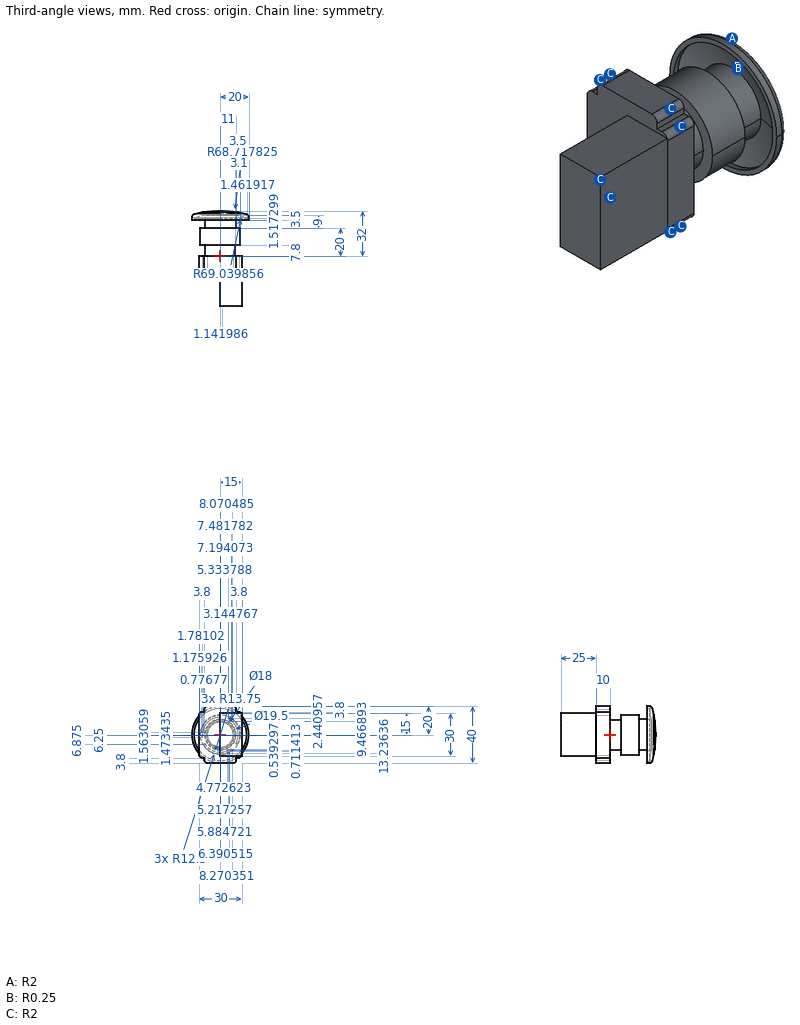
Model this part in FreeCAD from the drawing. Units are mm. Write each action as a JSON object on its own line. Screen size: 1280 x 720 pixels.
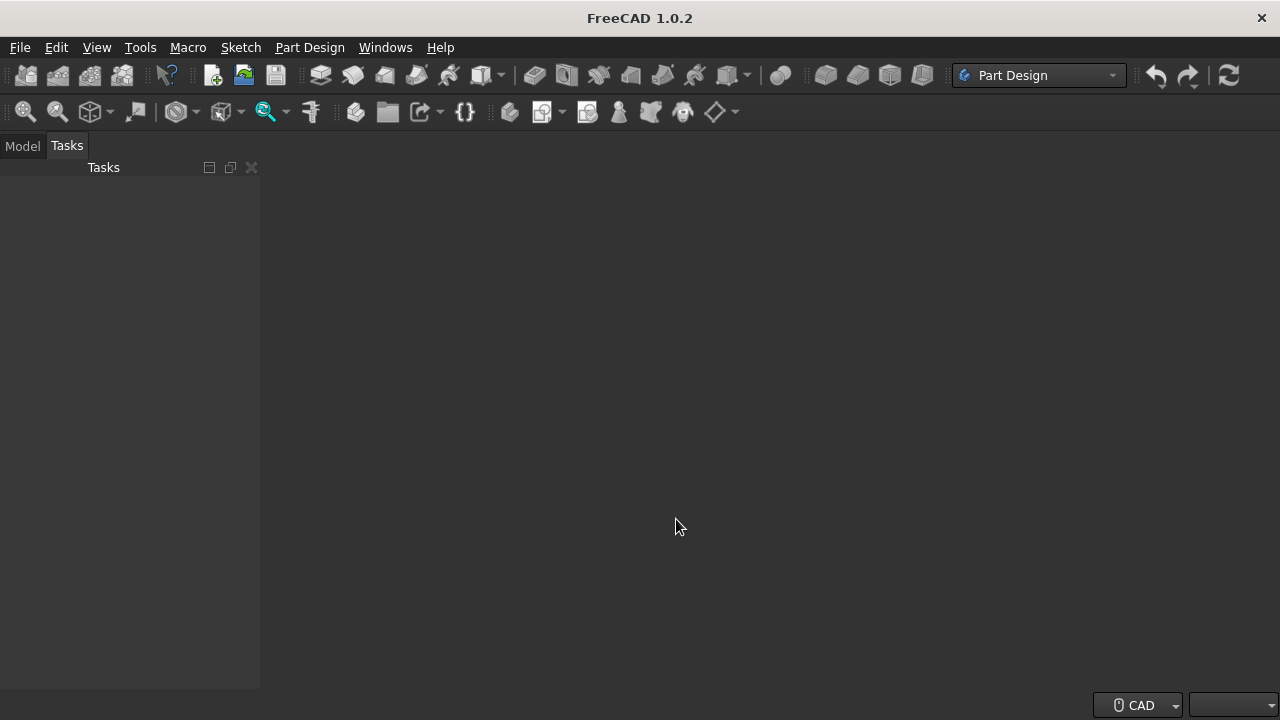
{"action": "left_click", "coordinate": [212, 76]}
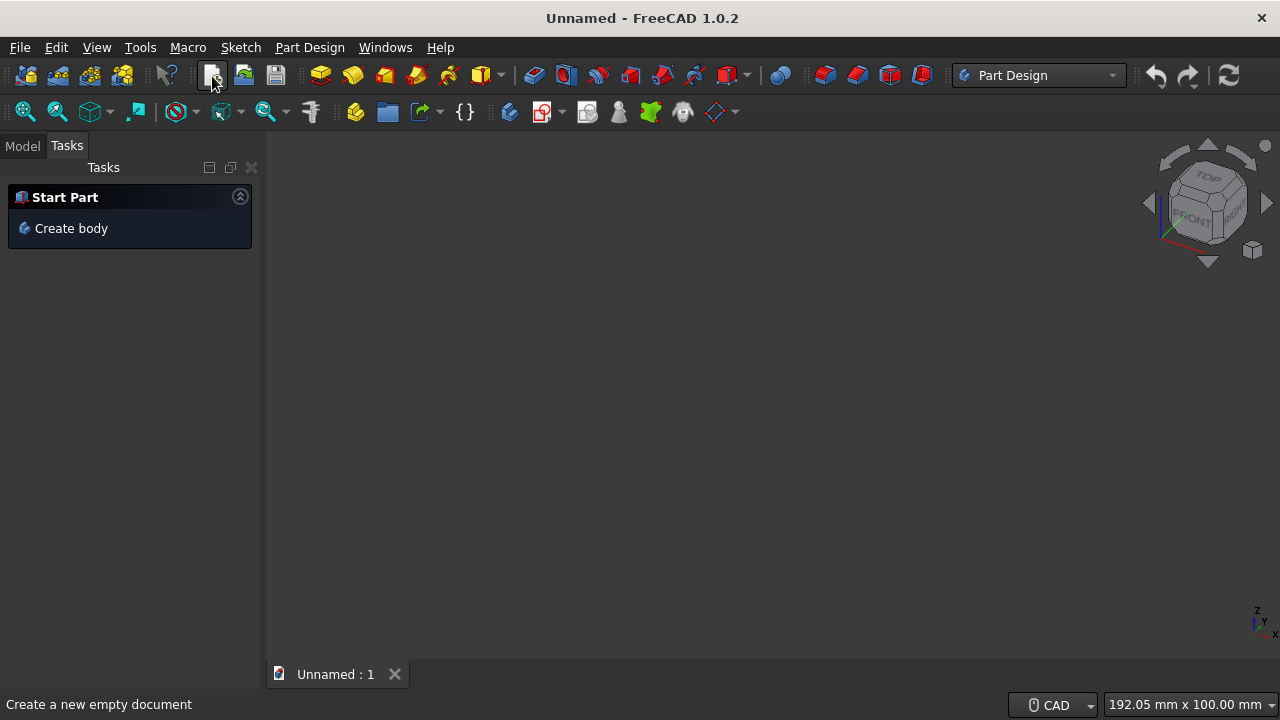
{"action": "left_click", "coordinate": [542, 112]}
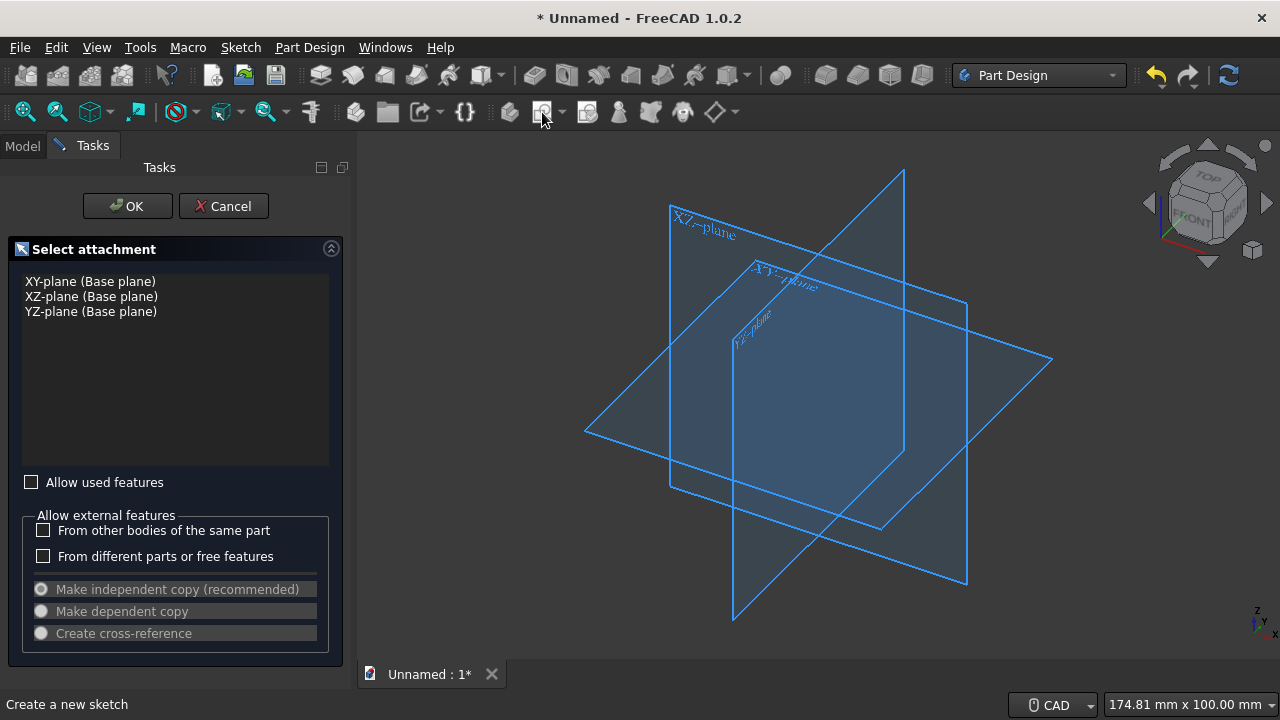
{"action": "left_click", "coordinate": [82, 282]}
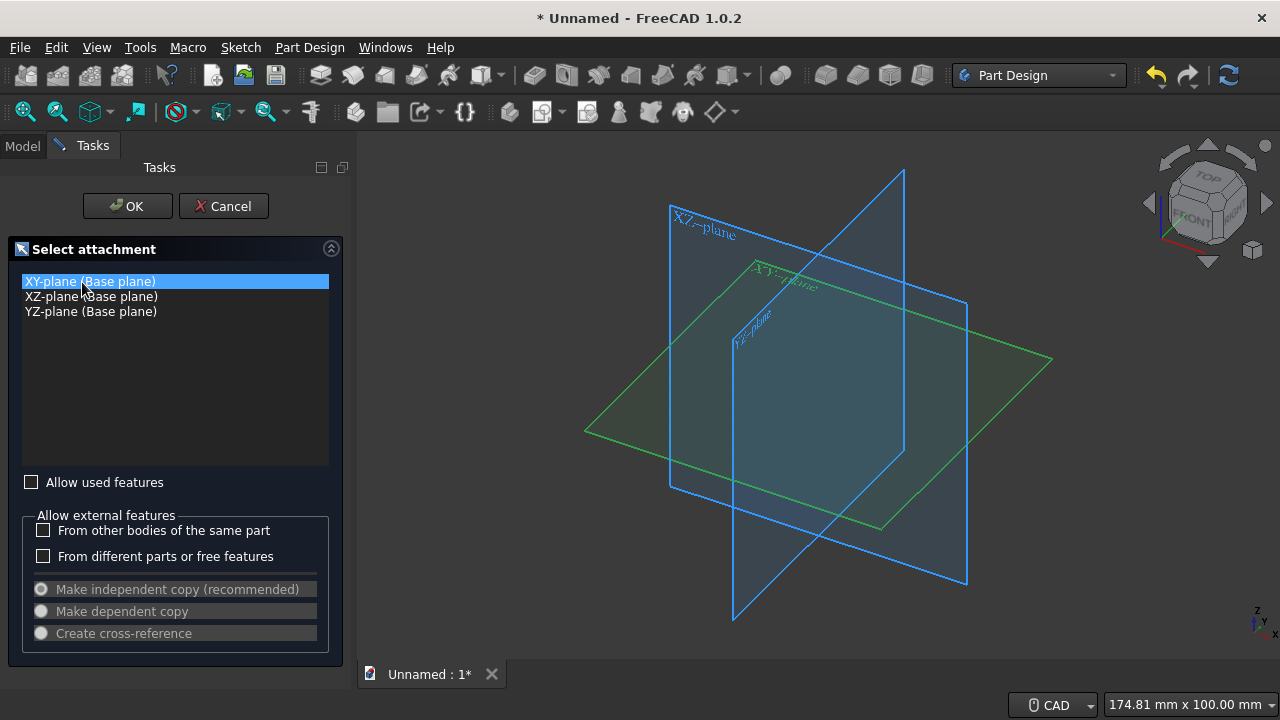
{"action": "left_click", "coordinate": [128, 206]}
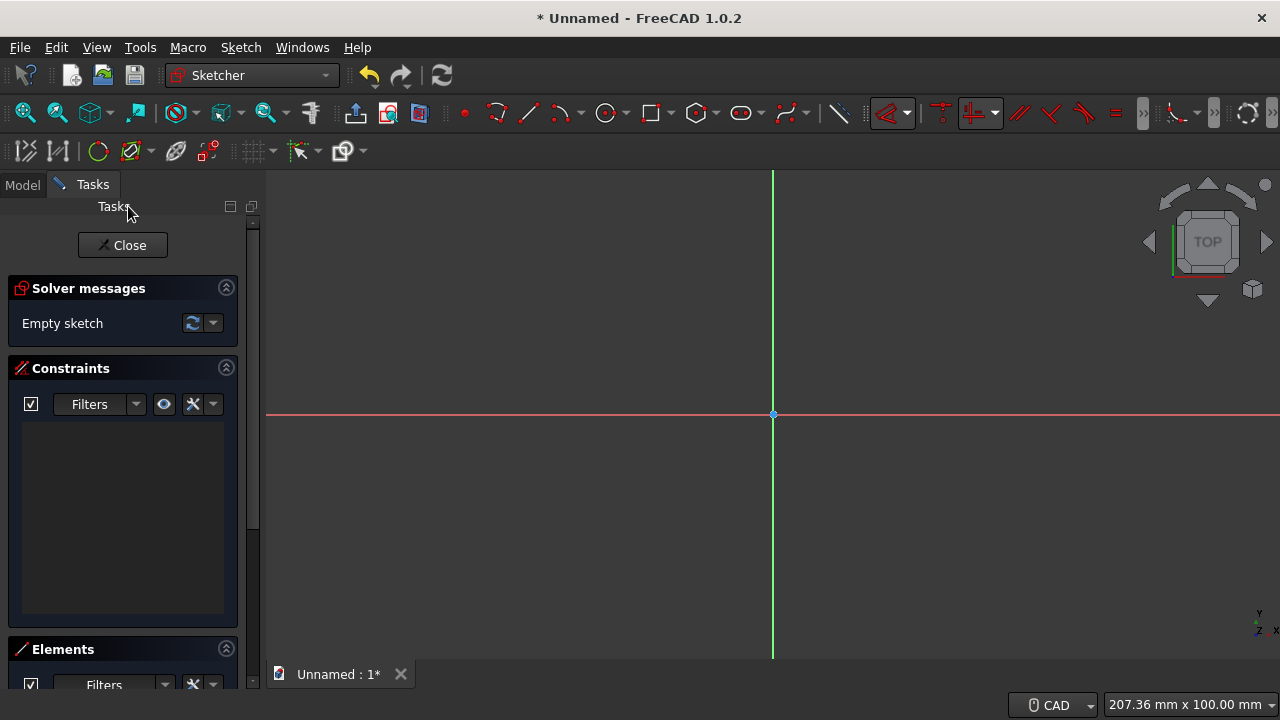
{"action": "scroll", "coordinate": [965, 241], "scroll_direction": "up", "scroll_amount": 3}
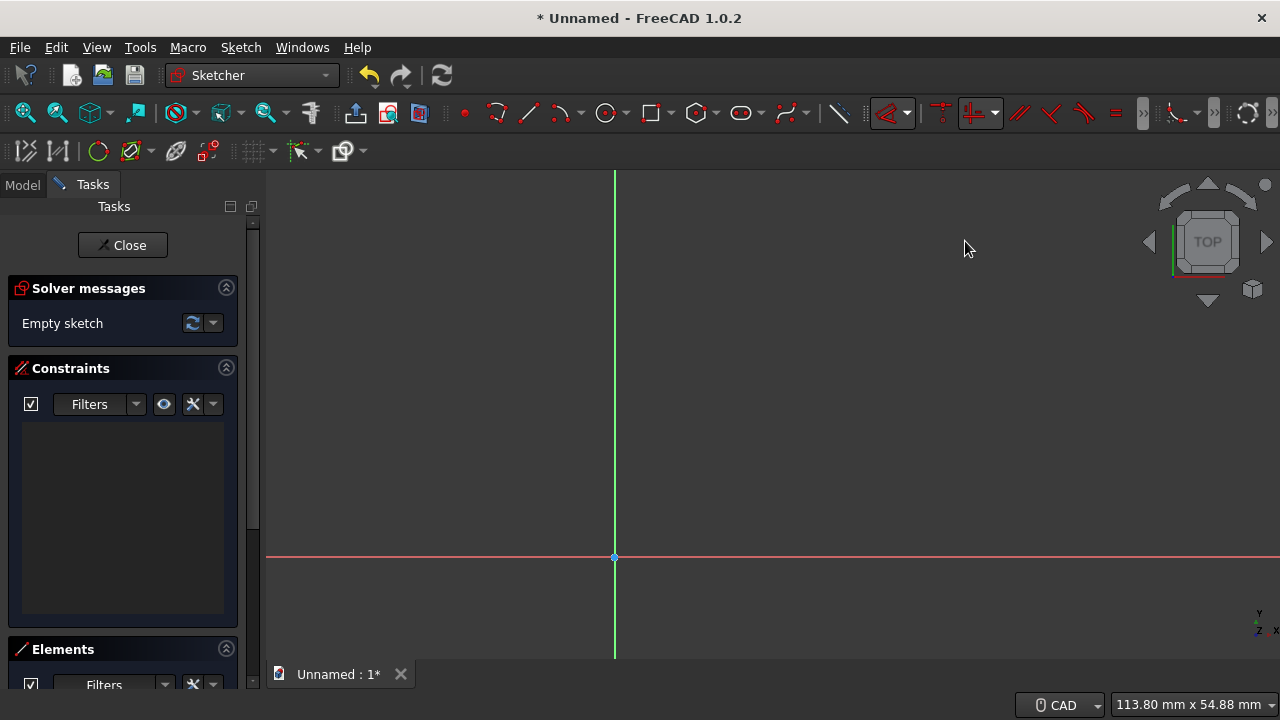
{"action": "left_click", "coordinate": [498, 114]}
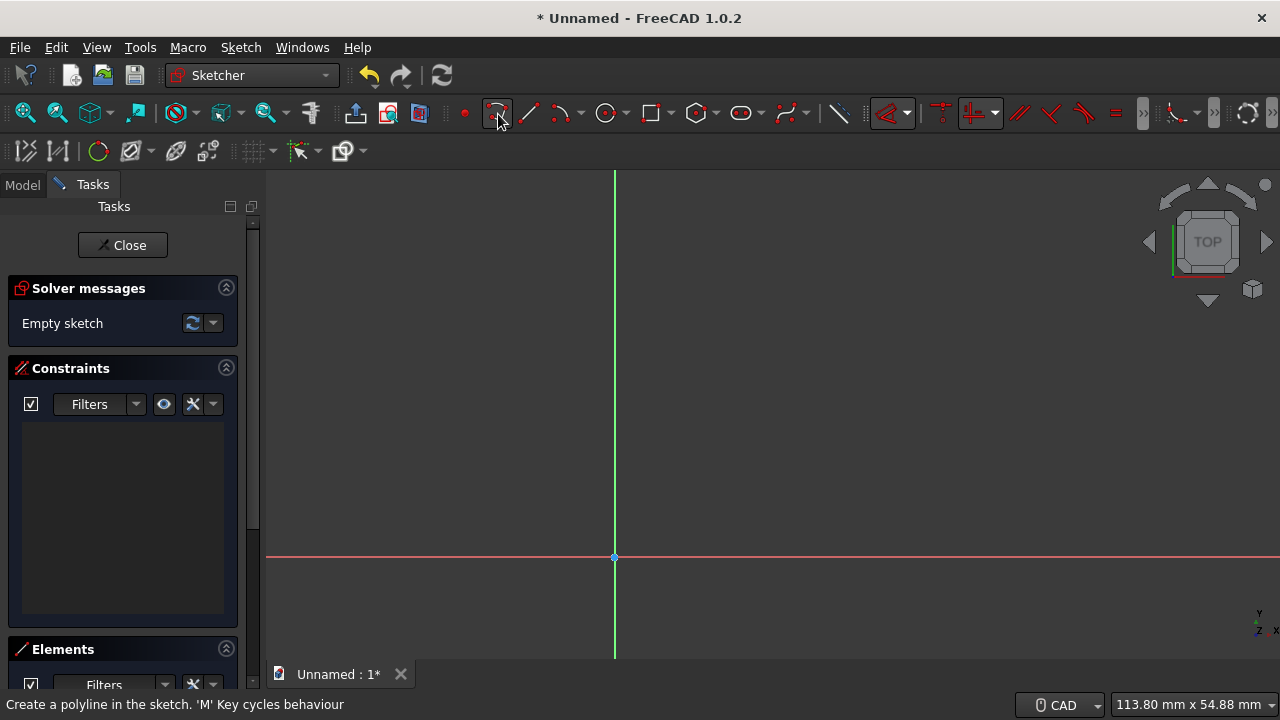
{"action": "left_click", "coordinate": [780, 313]}
{"action": "left_click", "coordinate": [780, 327]}
{"action": "left_click", "coordinate": [793, 327]}
{"action": "left_click", "coordinate": [793, 295]}
{"action": "right_click", "coordinate": [793, 295]}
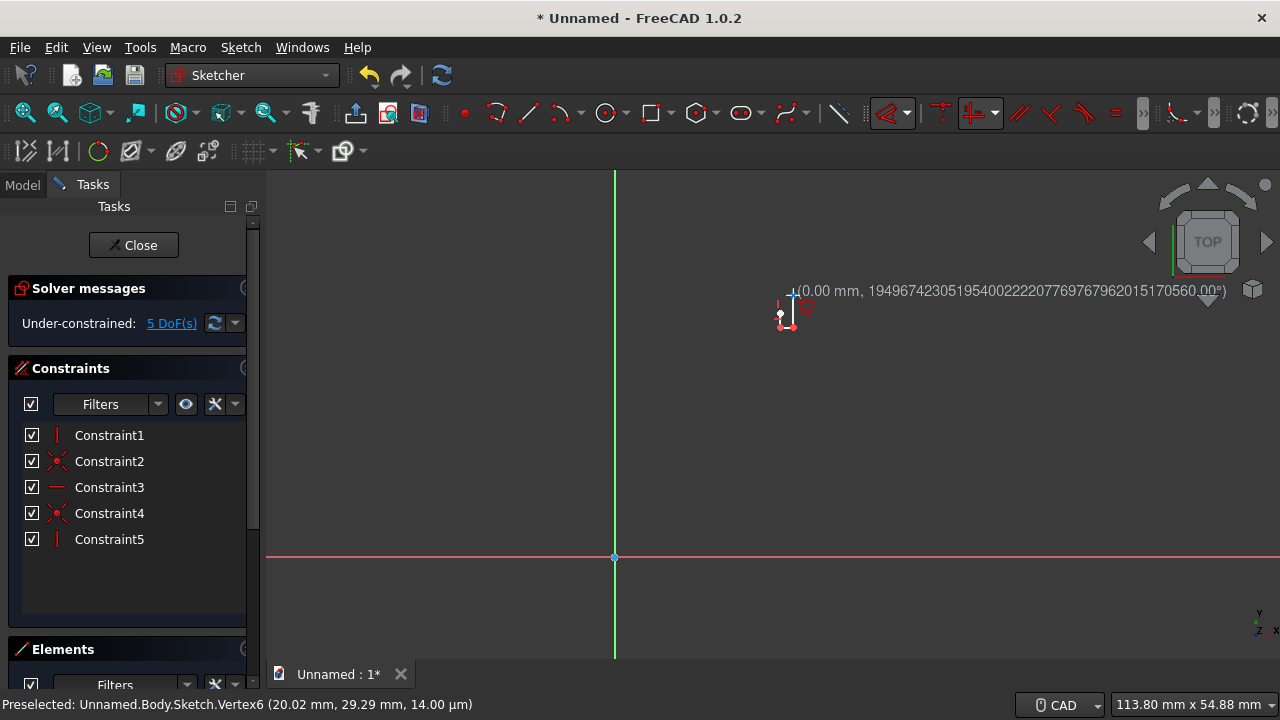
{"action": "left_click", "coordinate": [615, 272]}
{"action": "left_click", "coordinate": [615, 557]}
{"action": "left_click", "coordinate": [709, 548]}
{"action": "left_click", "coordinate": [709, 488]}
{"action": "left_click", "coordinate": [740, 488]}
{"action": "left_click", "coordinate": [740, 379]}
{"action": "left_click", "coordinate": [713, 379]}
{"action": "left_click", "coordinate": [713, 299]}
{"action": "right_click", "coordinate": [713, 299]}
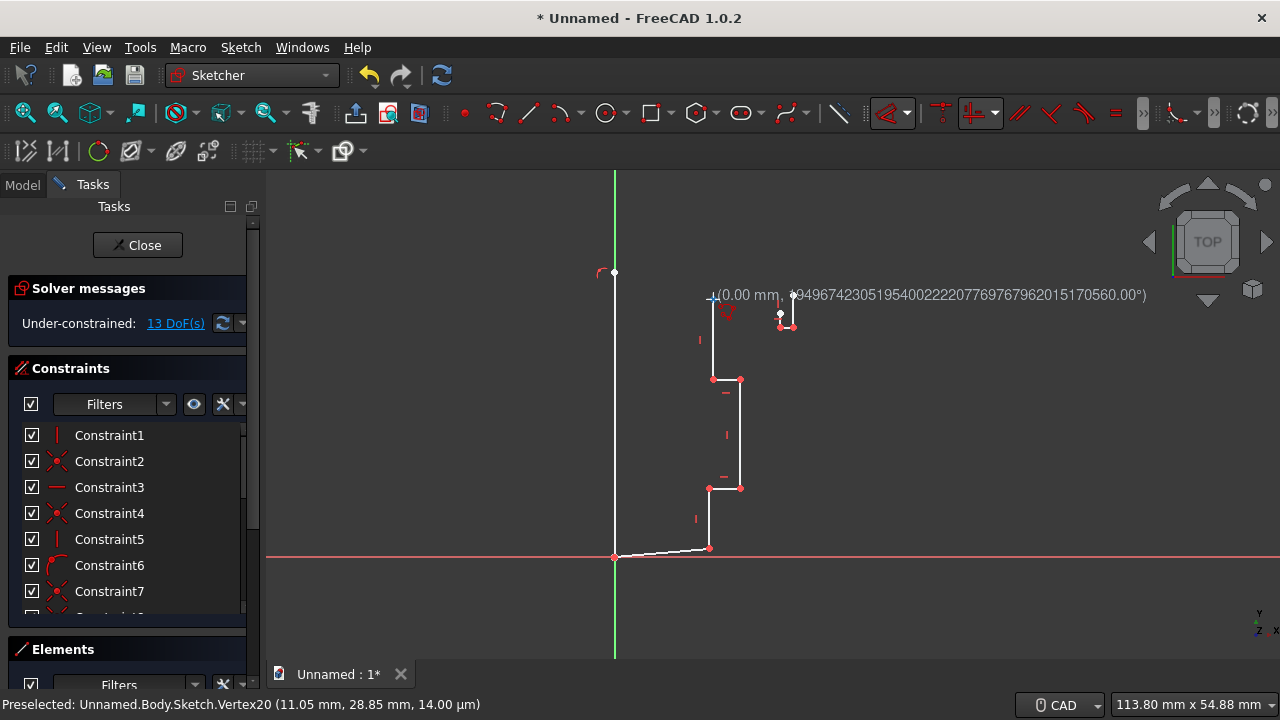
{"action": "left_click", "coordinate": [584, 114]}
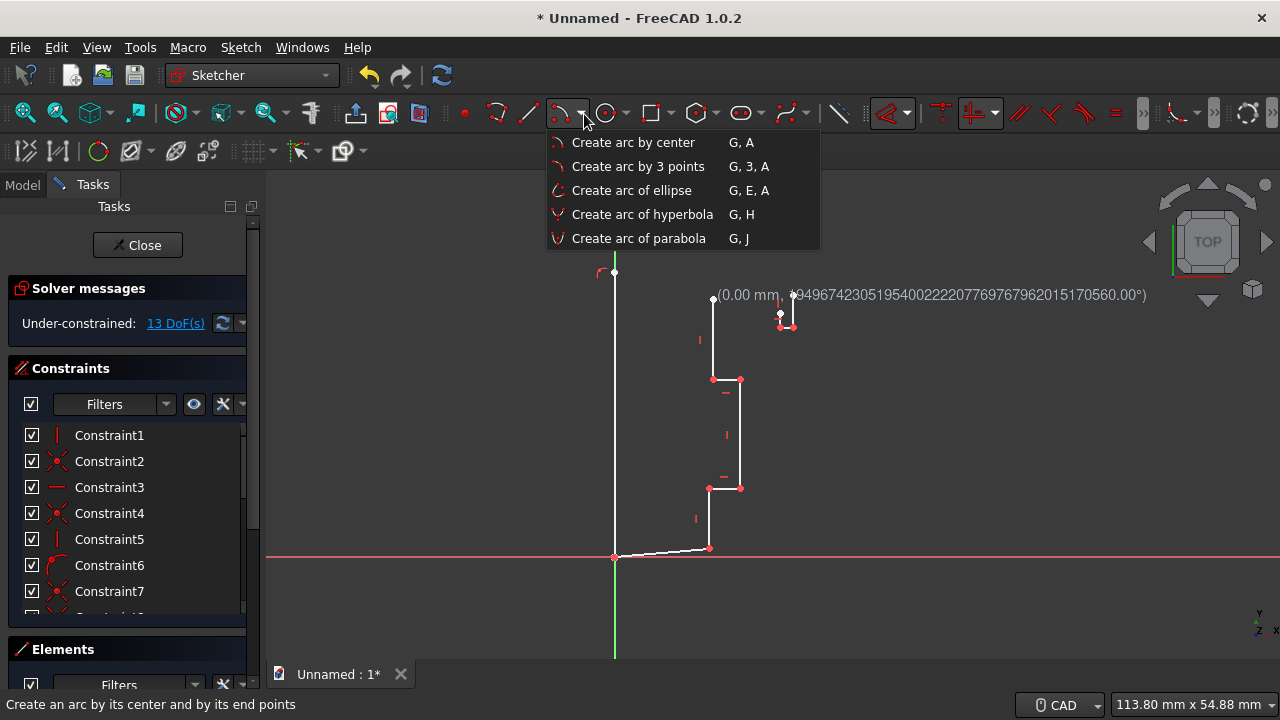
{"action": "left_click", "coordinate": [684, 166]}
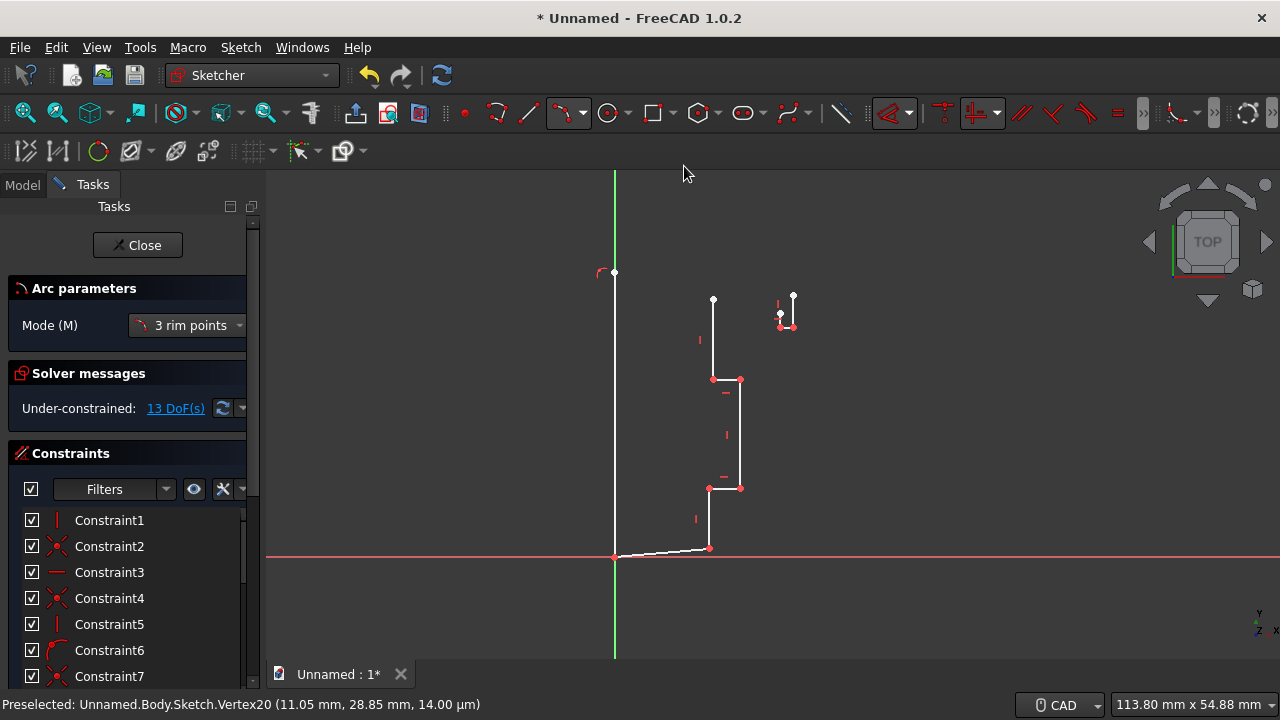
{"action": "left_click", "coordinate": [793, 296]}
{"action": "left_click", "coordinate": [615, 273]}